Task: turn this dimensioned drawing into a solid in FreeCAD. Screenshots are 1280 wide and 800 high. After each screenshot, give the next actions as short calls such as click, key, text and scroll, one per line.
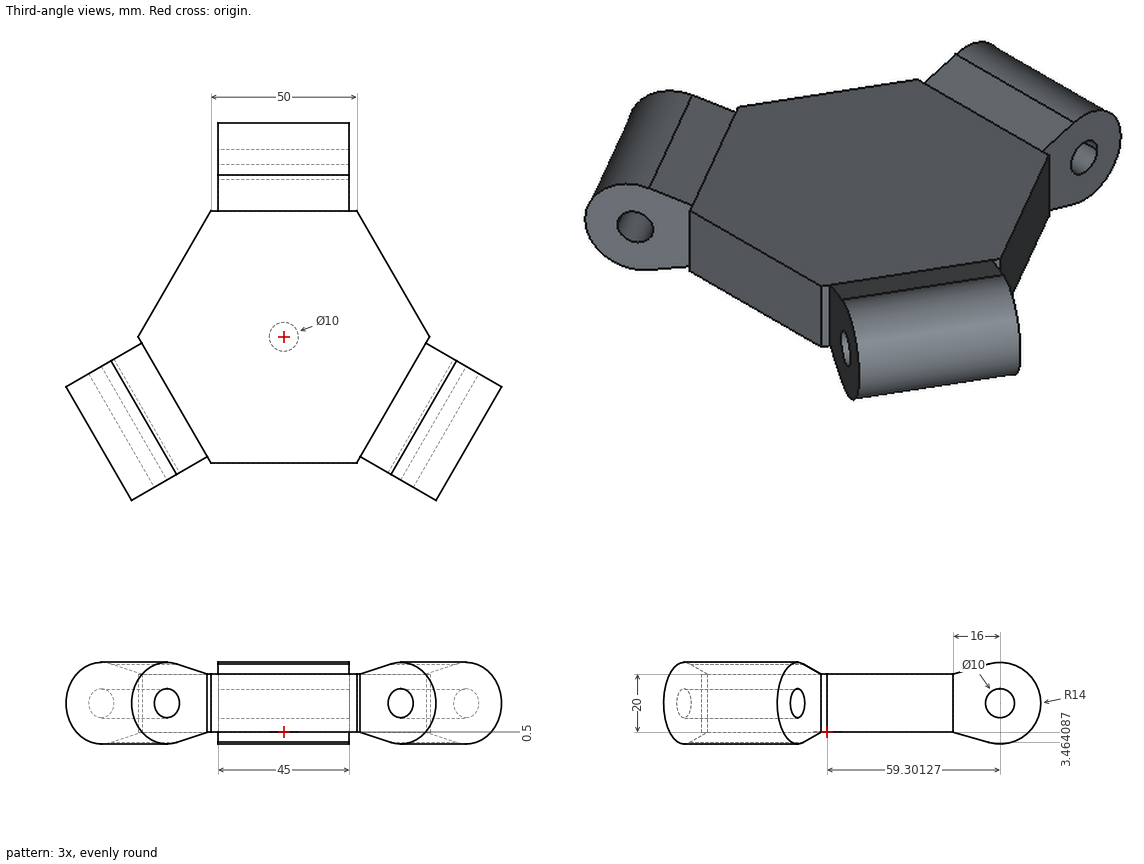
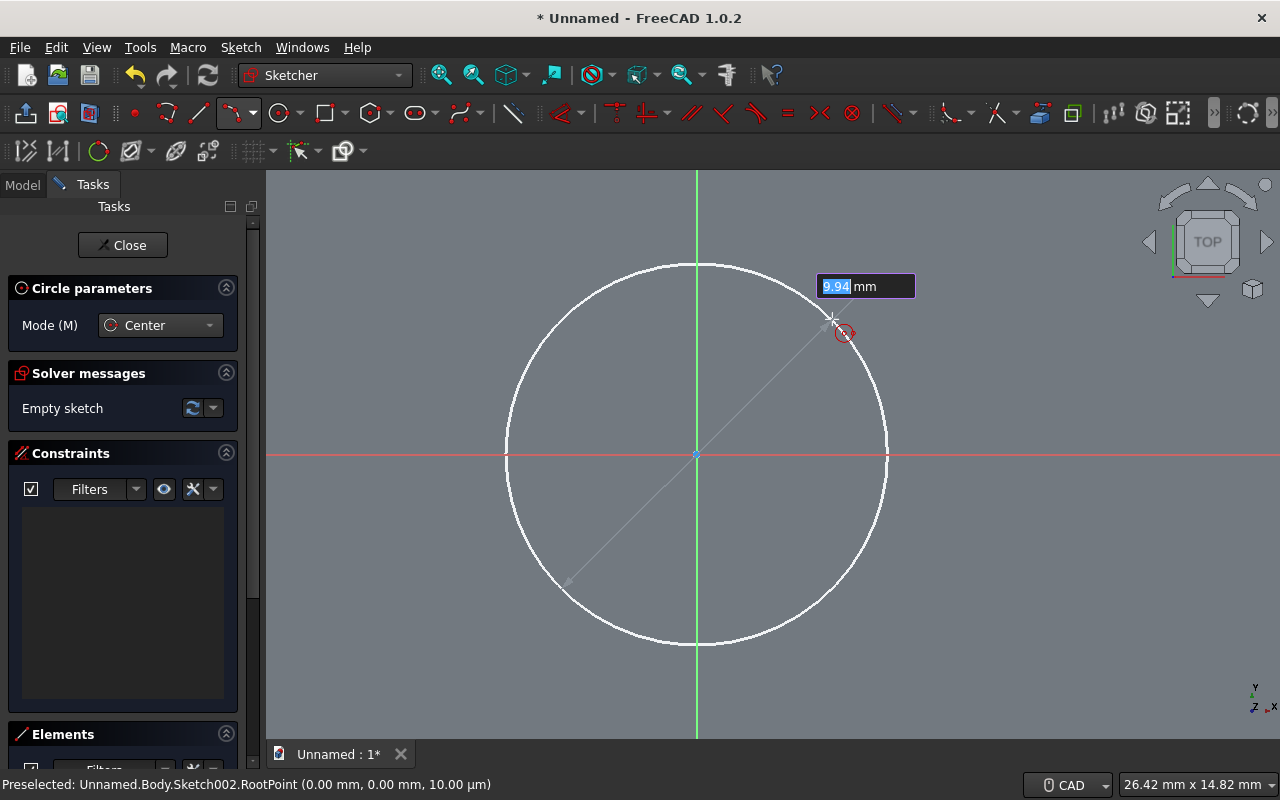
text(10)
key(Return)
key(Escape)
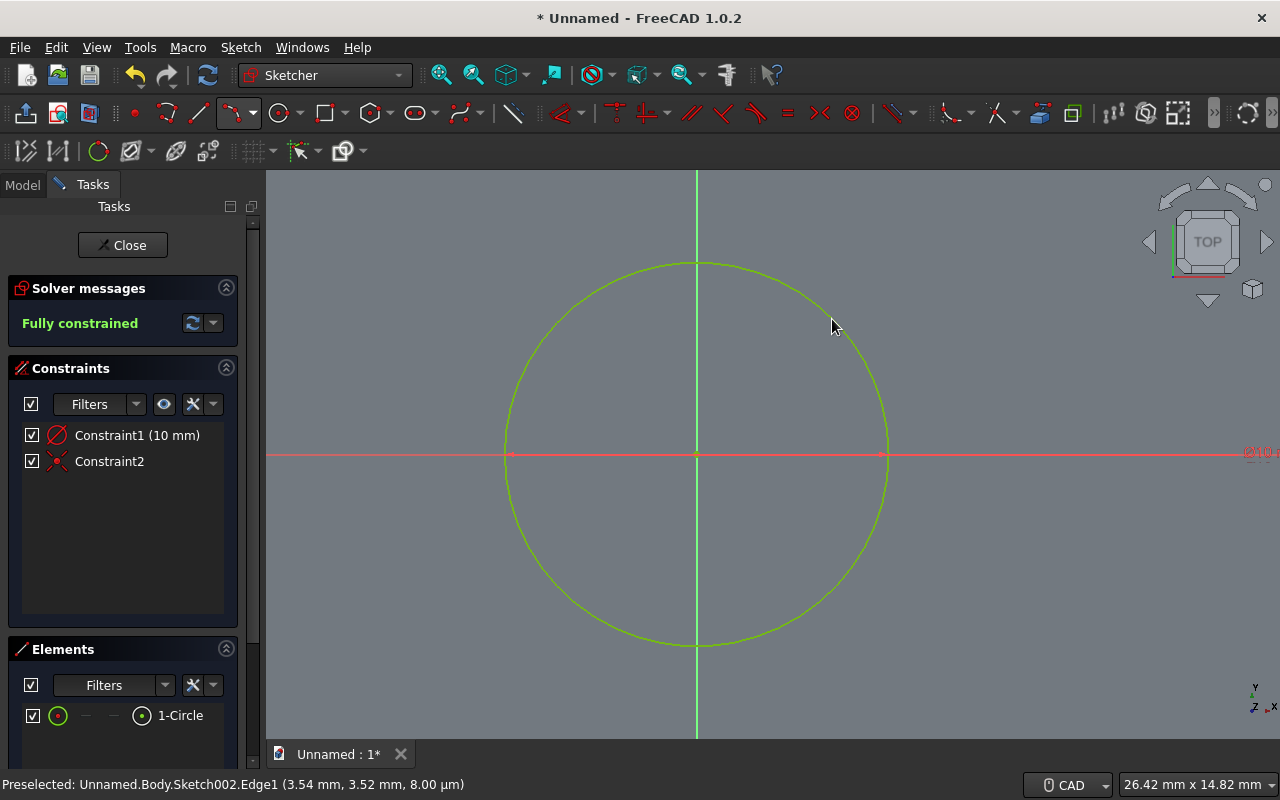
click(123, 245)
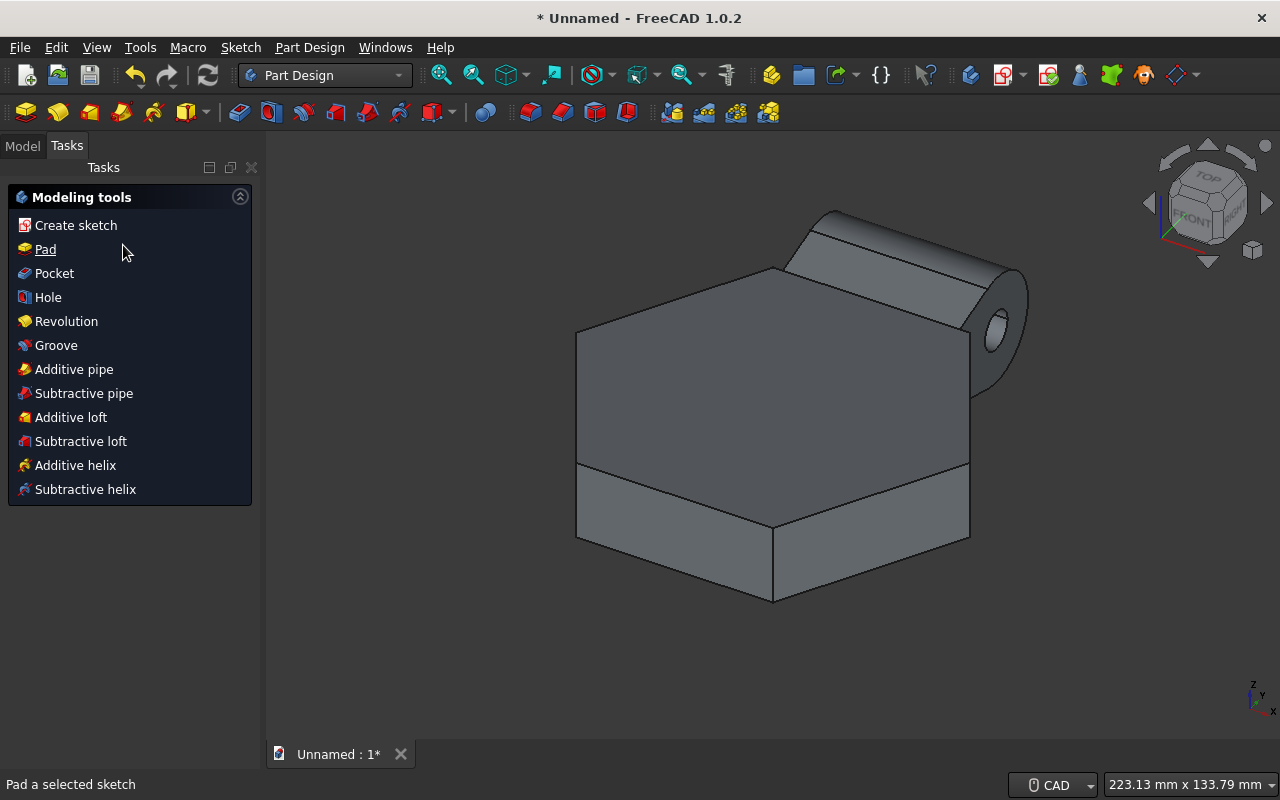
click(240, 112)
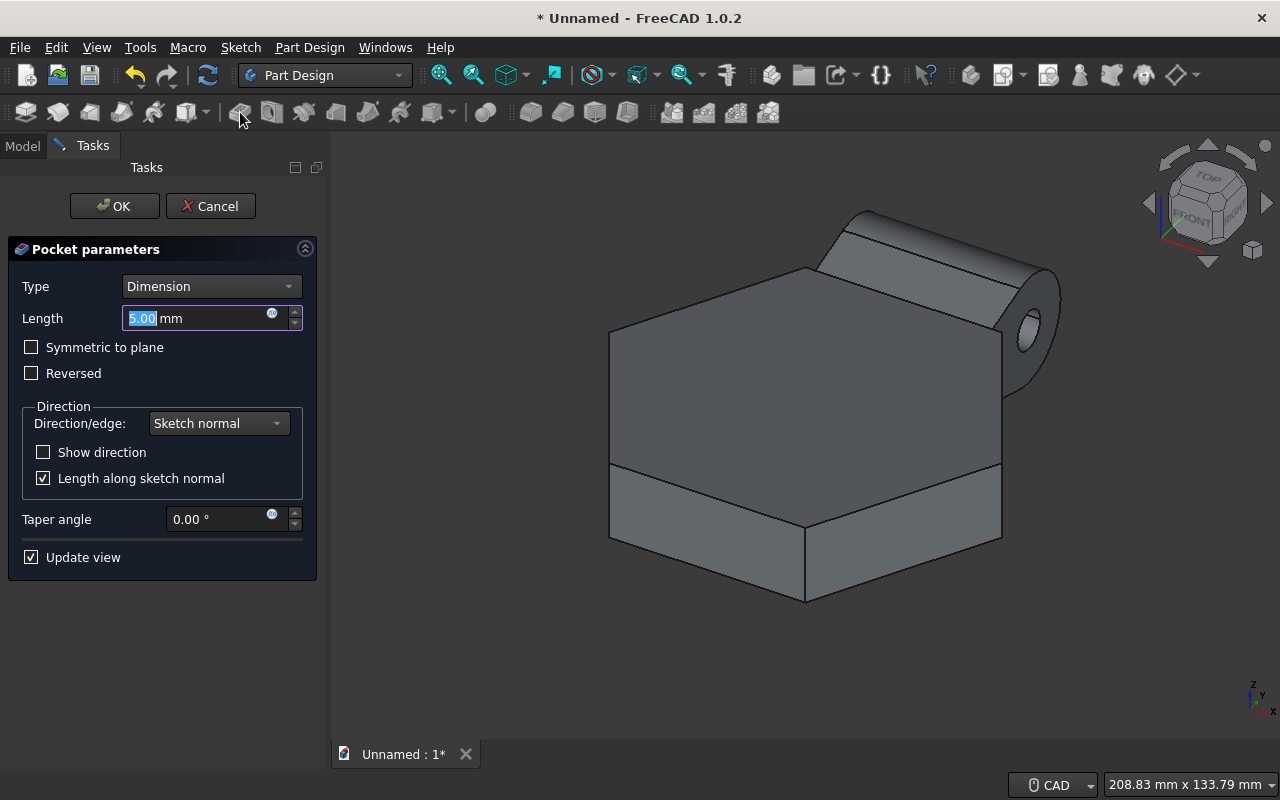
text(0.5)
key(Tab)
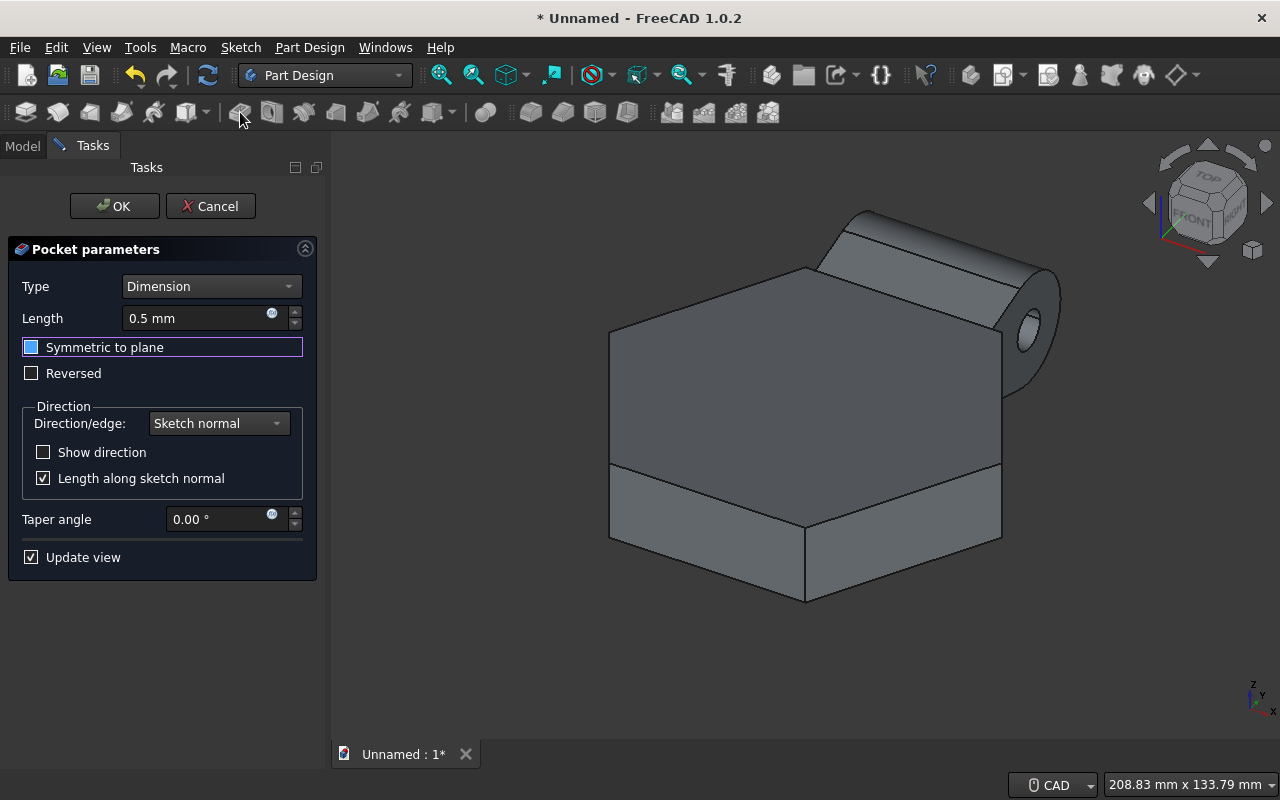
click(30, 373)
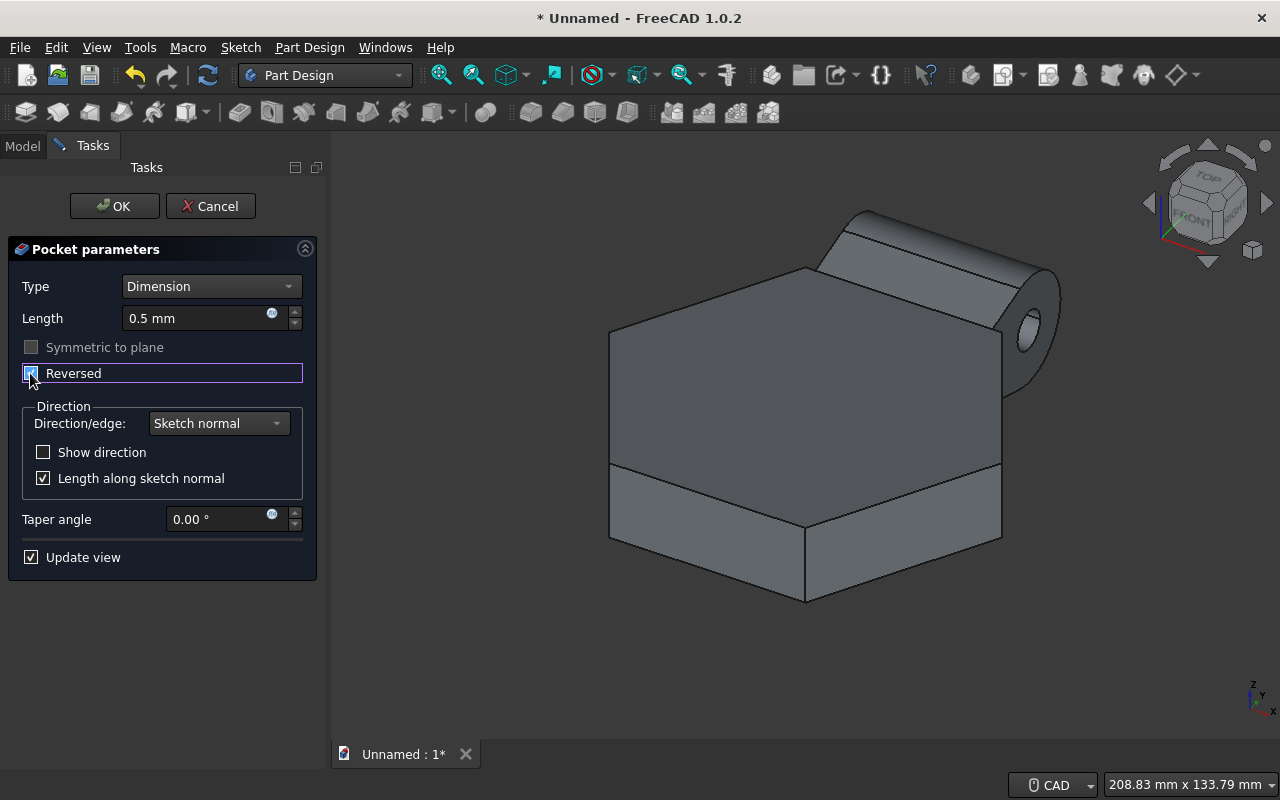
click(115, 206)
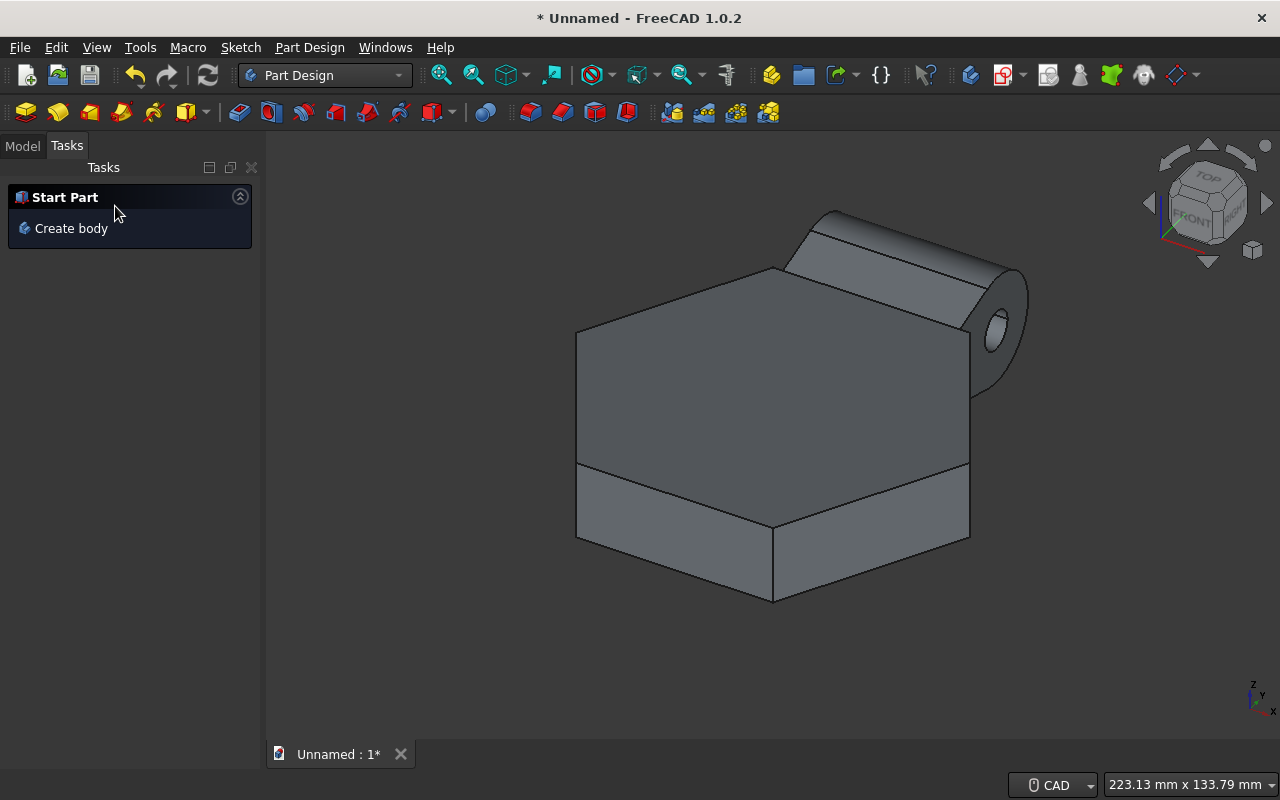
click(23, 145)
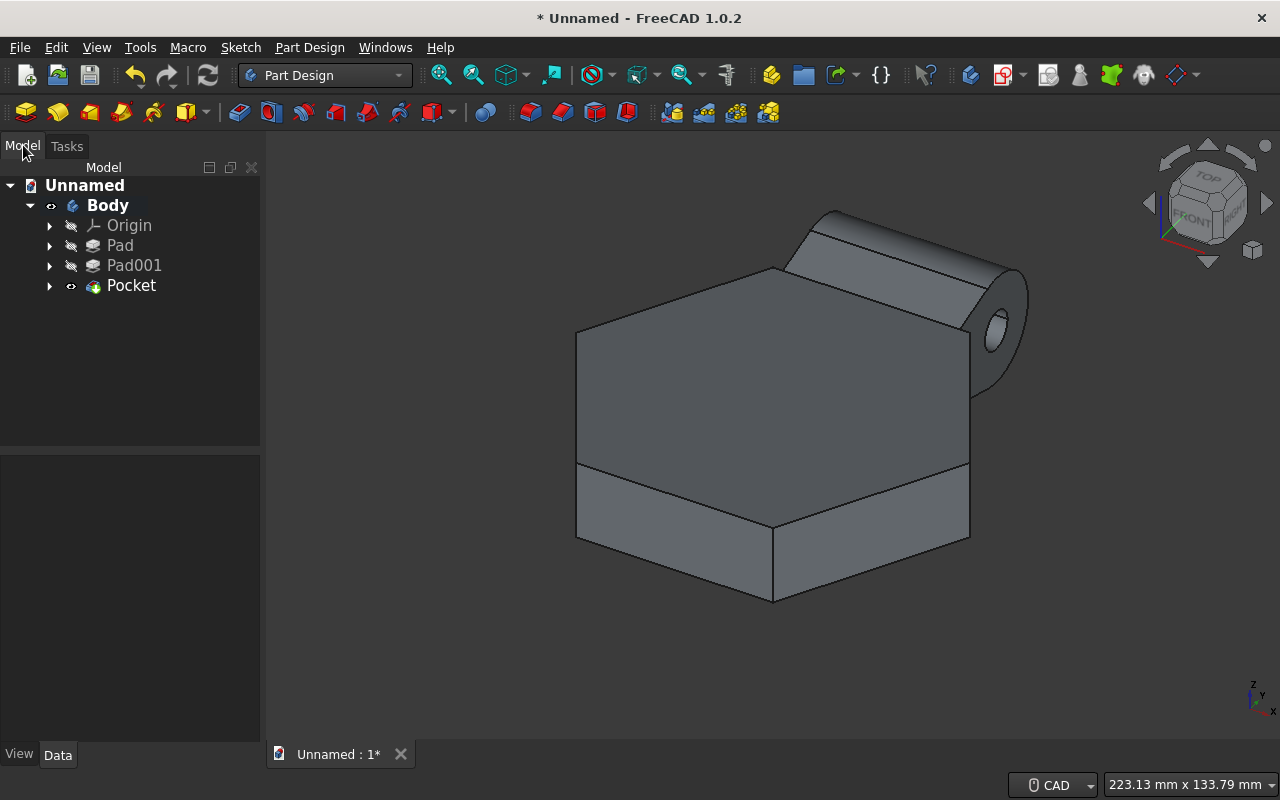
click(116, 266)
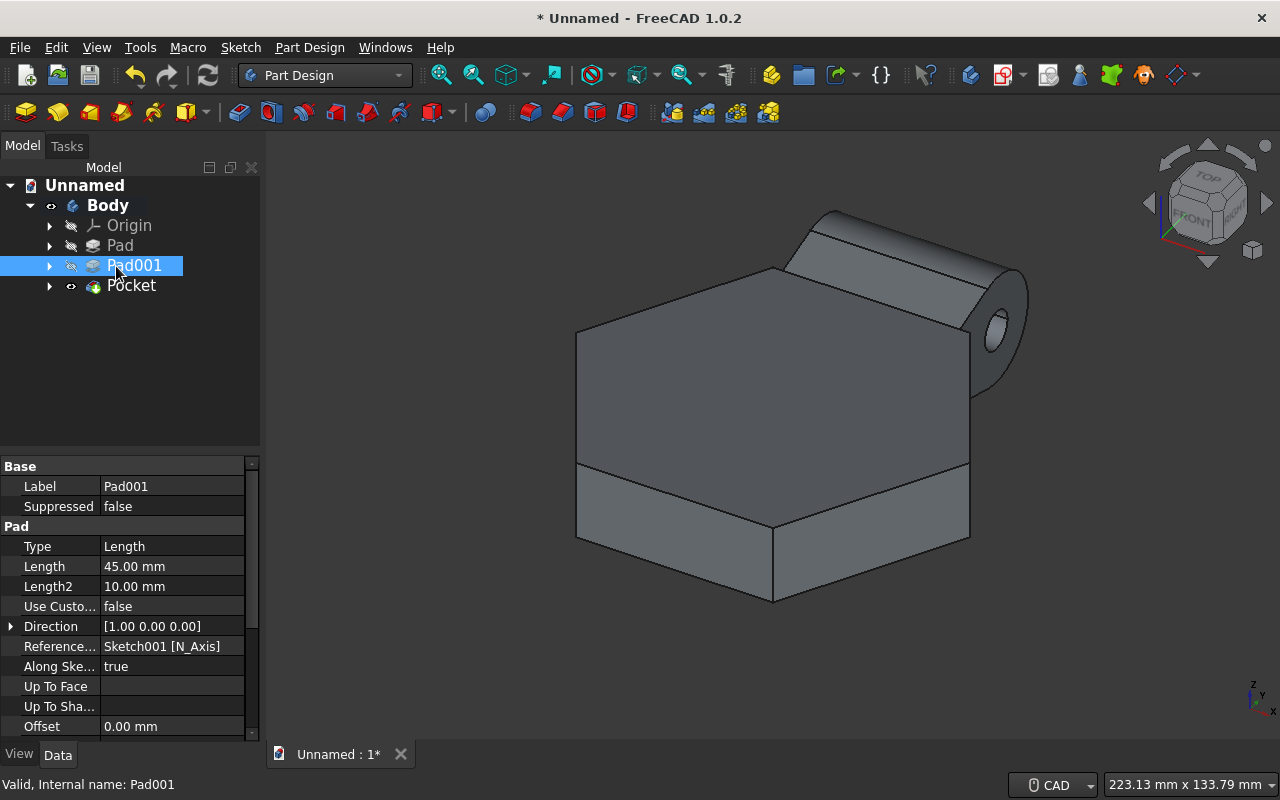
click(736, 112)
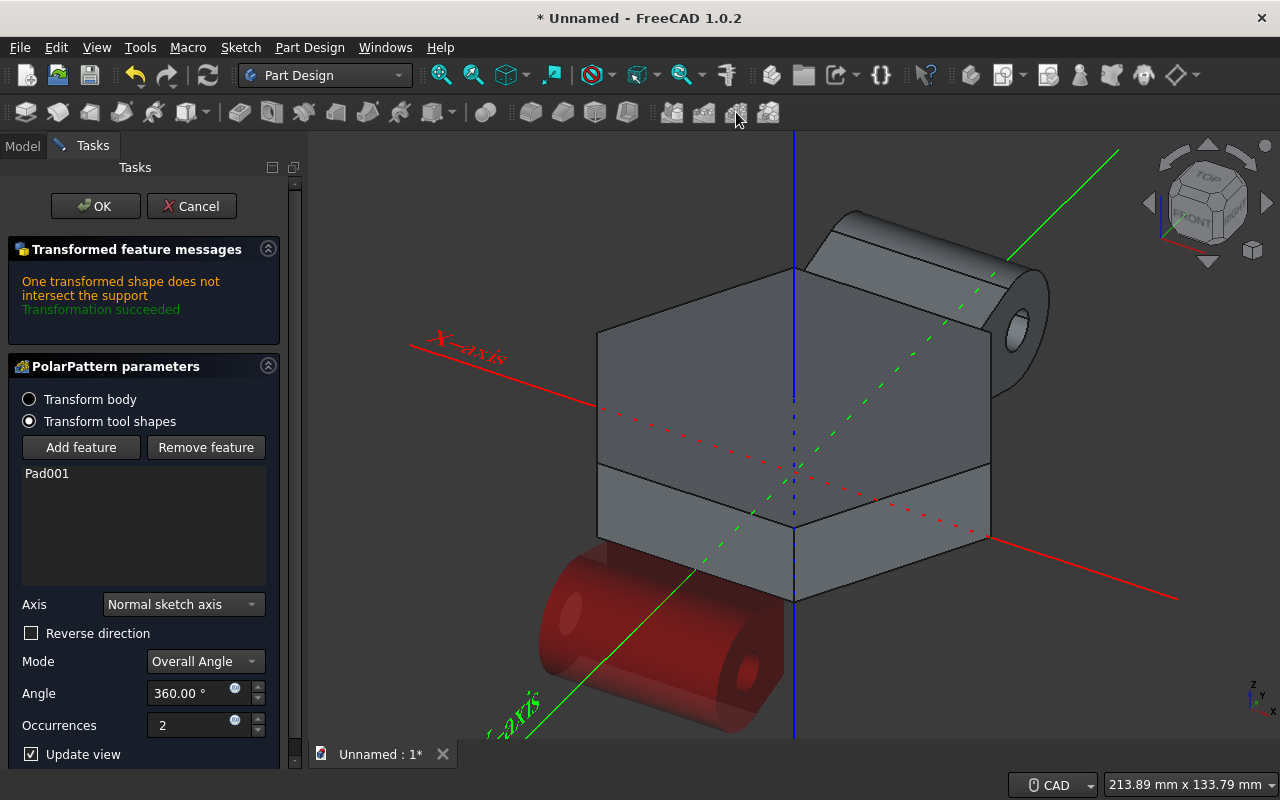
click(184, 604)